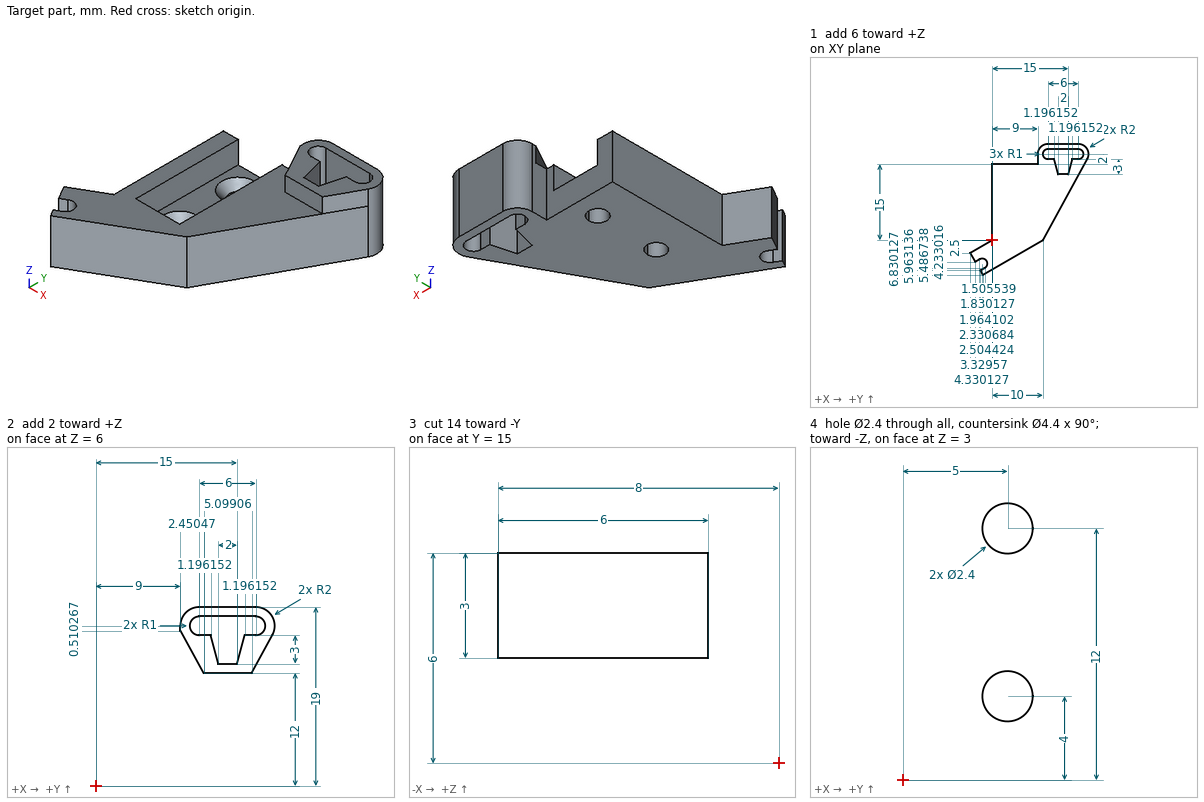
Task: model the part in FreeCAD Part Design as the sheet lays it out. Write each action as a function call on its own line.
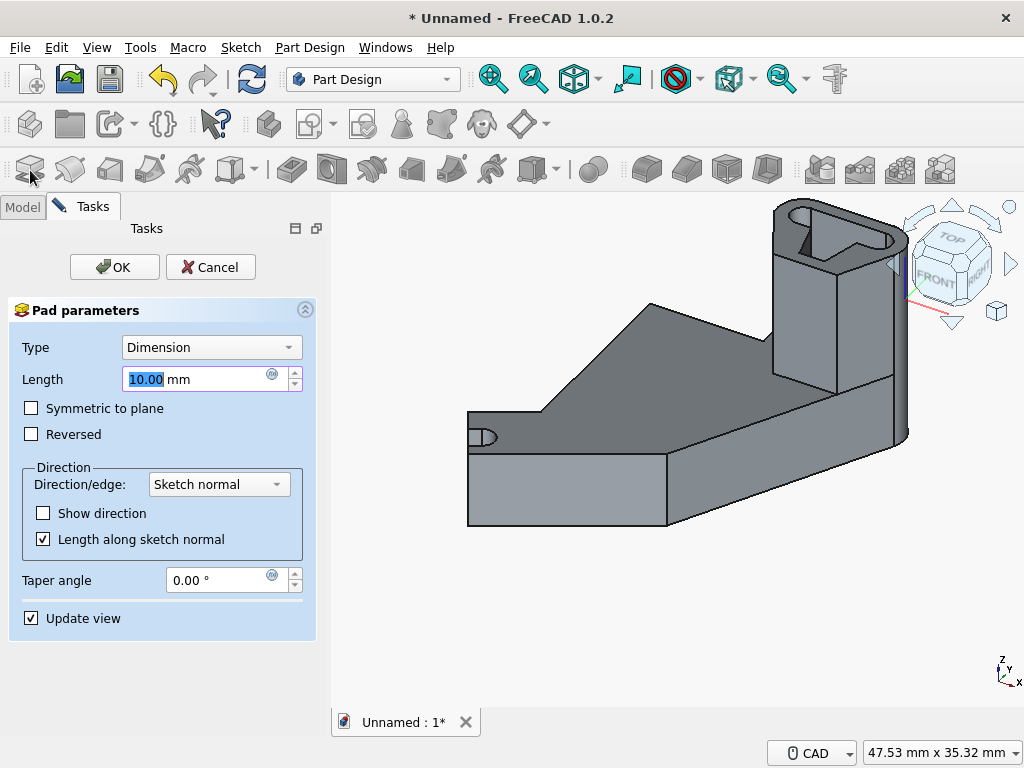
text(2)
key(Tab)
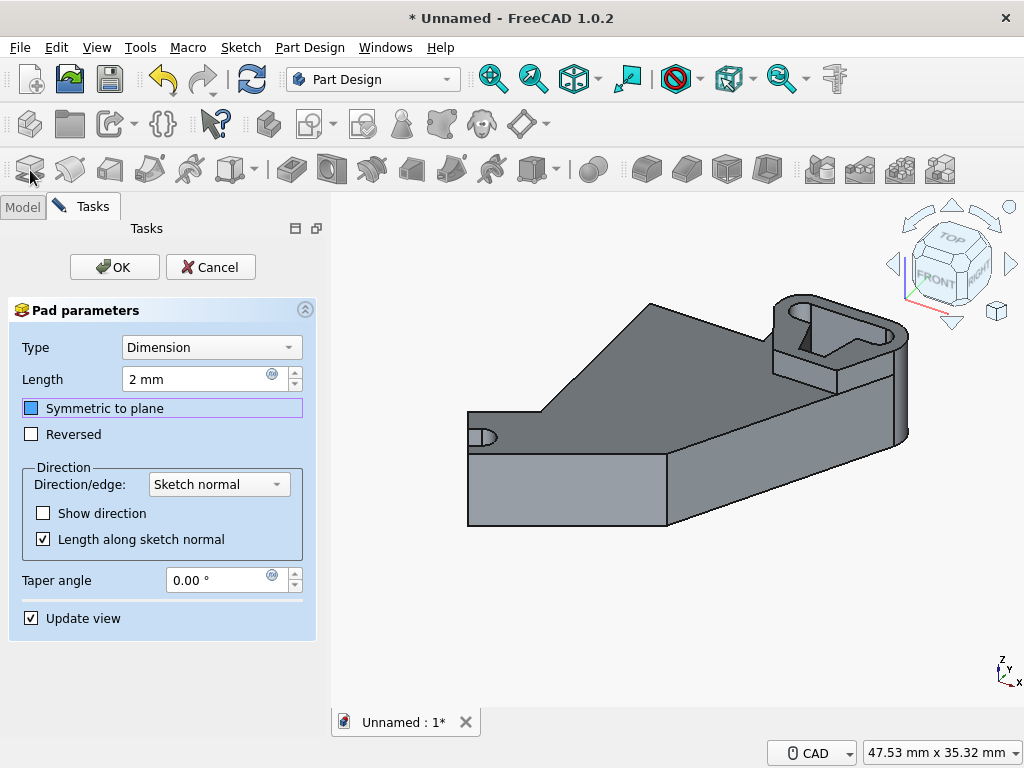
click(115, 267)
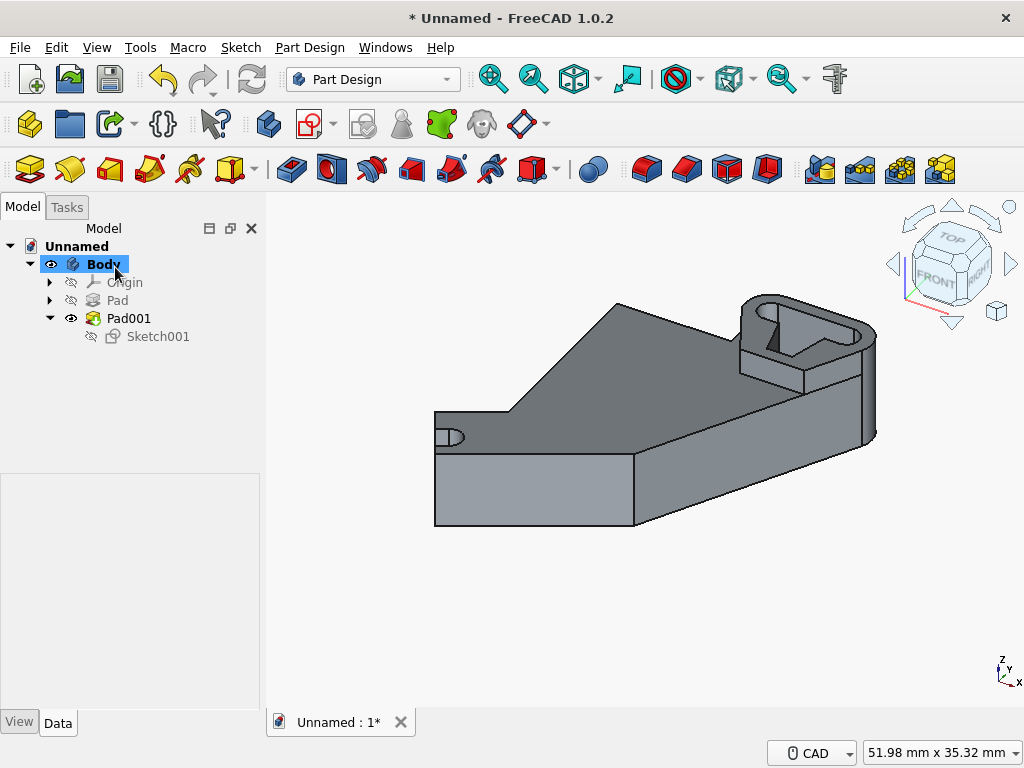
key(4)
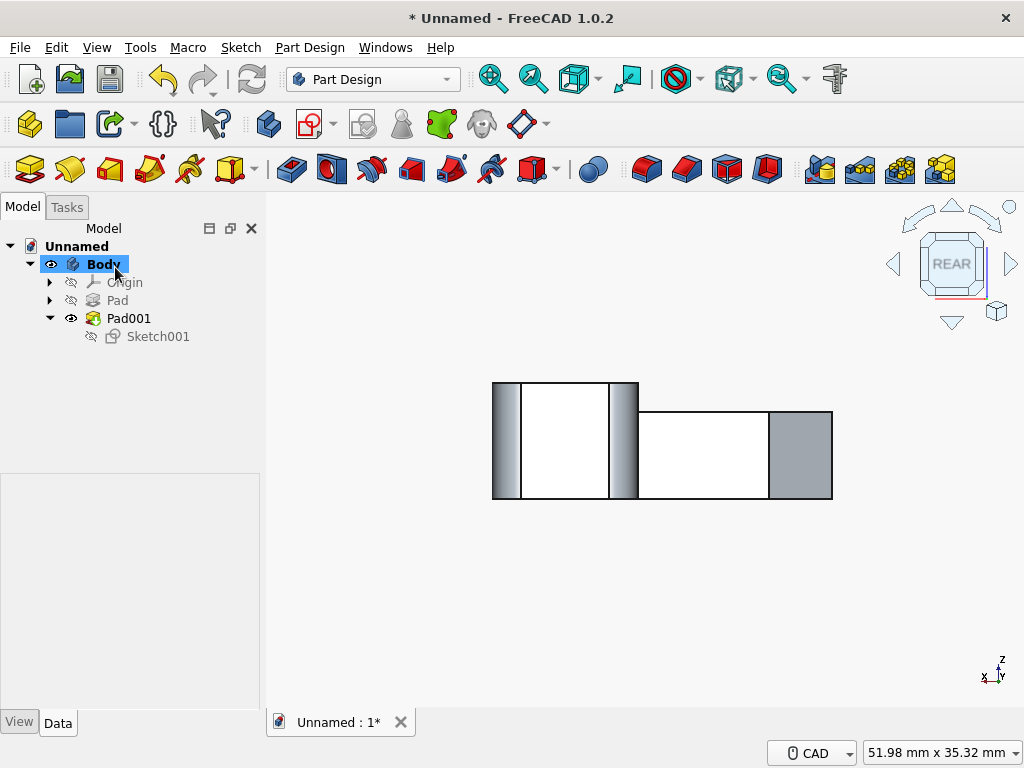
key(v)
key(f)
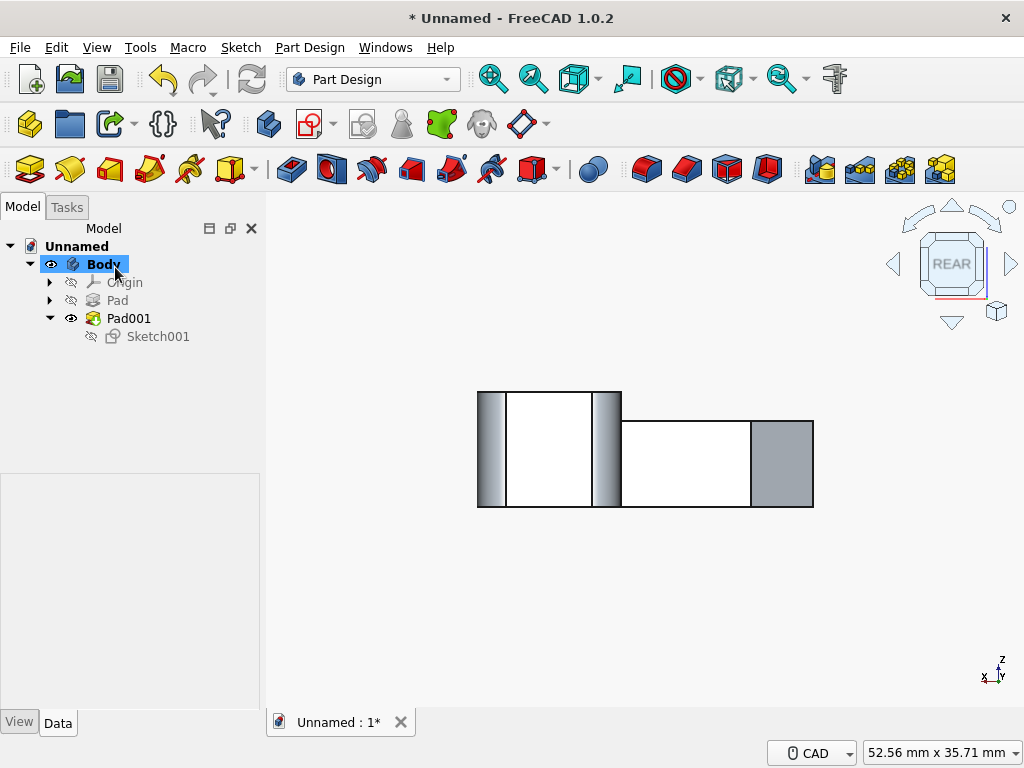
click(667, 463)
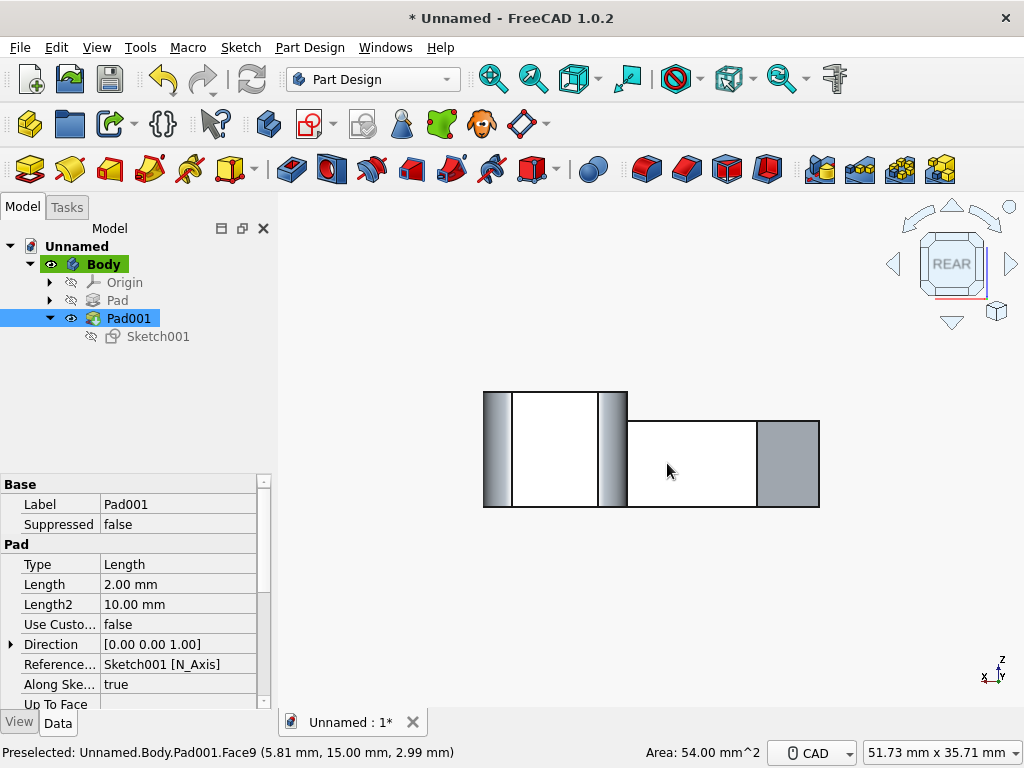
click(310, 124)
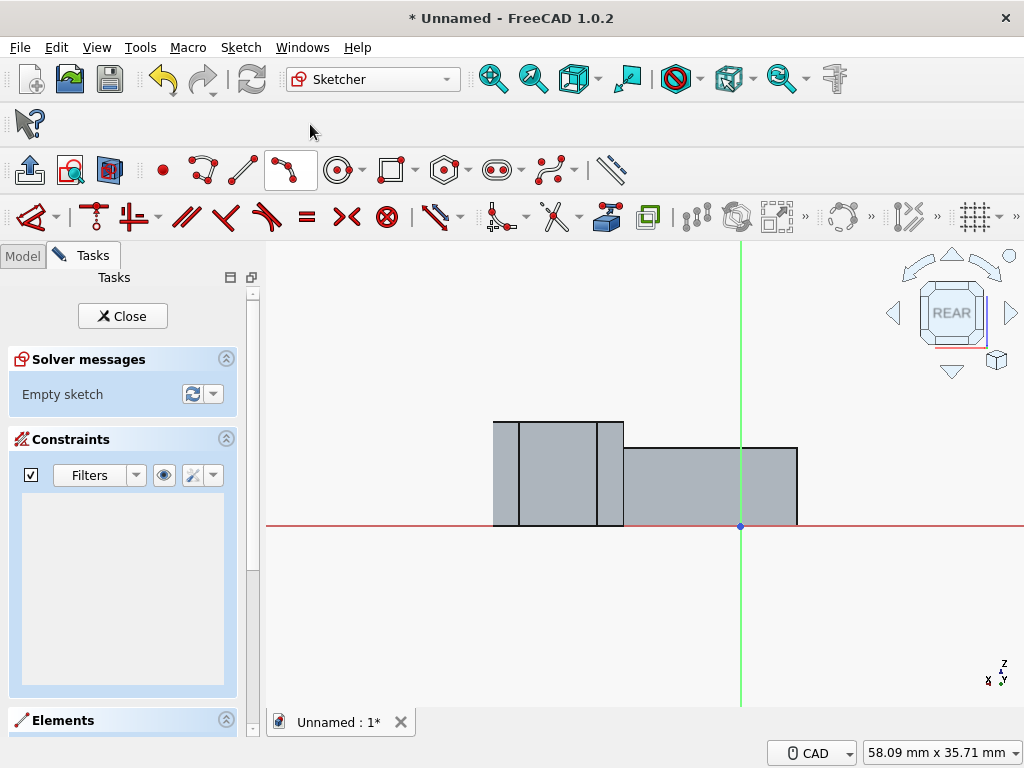
scroll(725, 491, up, 7)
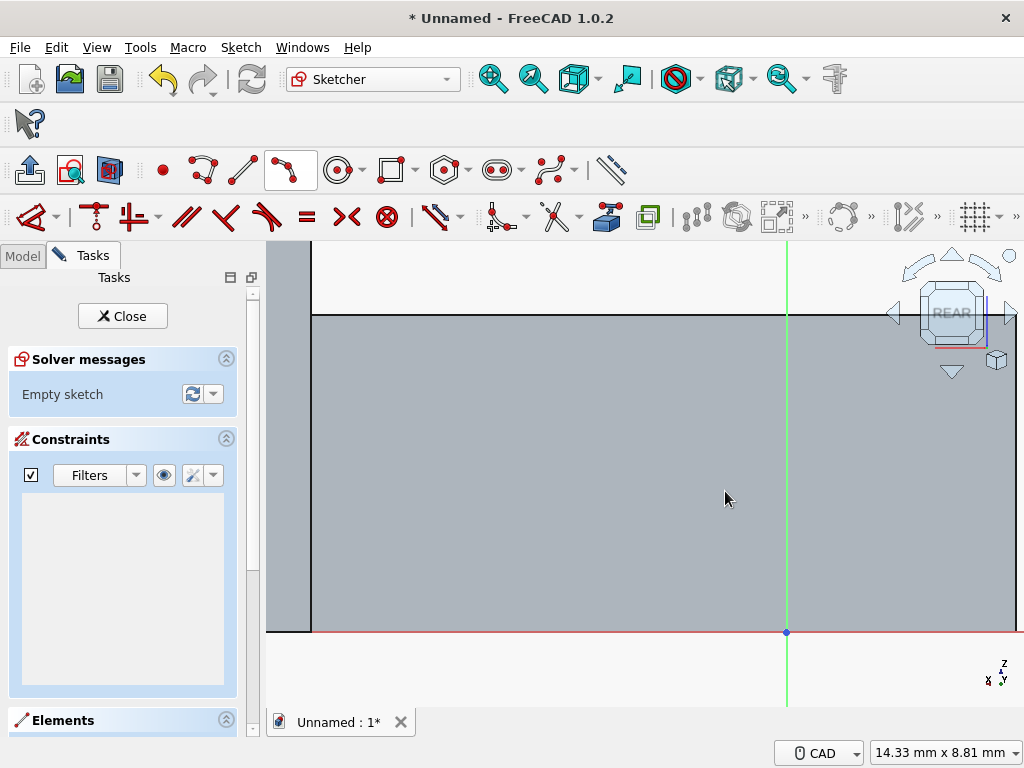
key(g)
key(r)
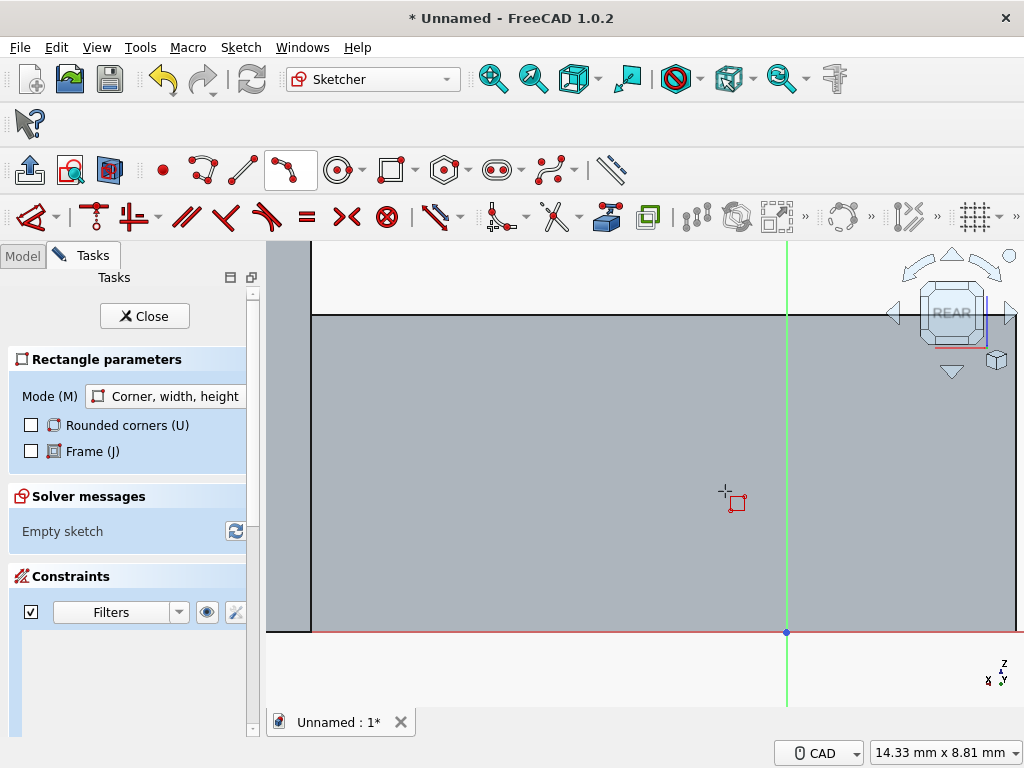
click(363, 315)
click(681, 473)
key(Escape)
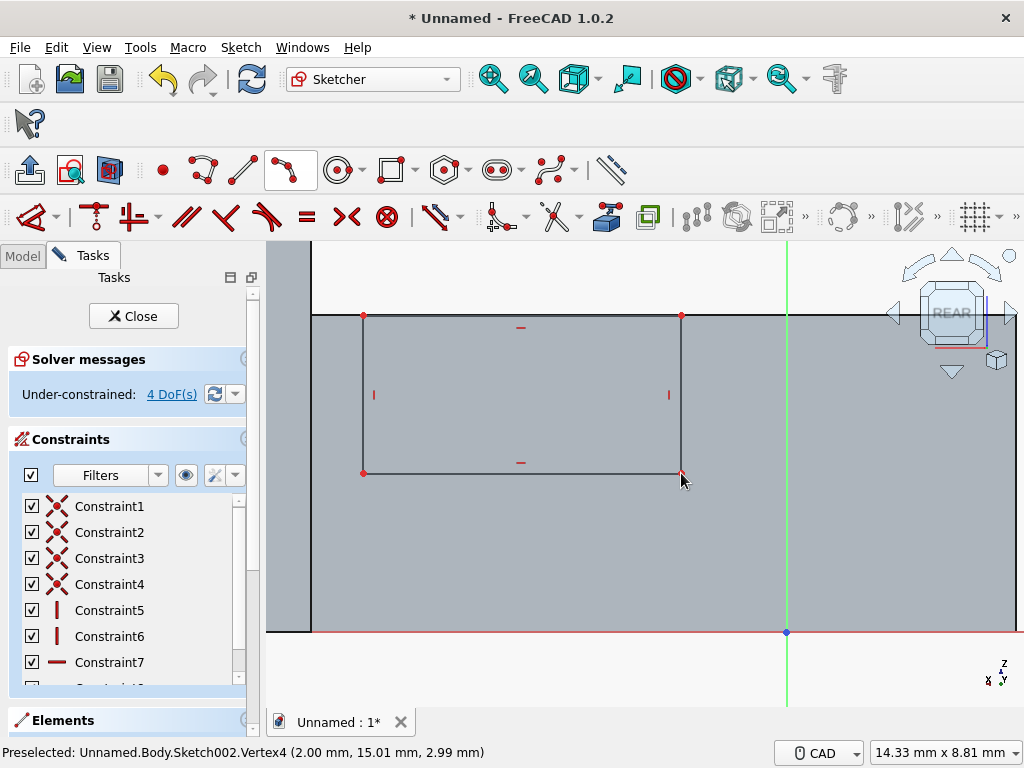
key(d)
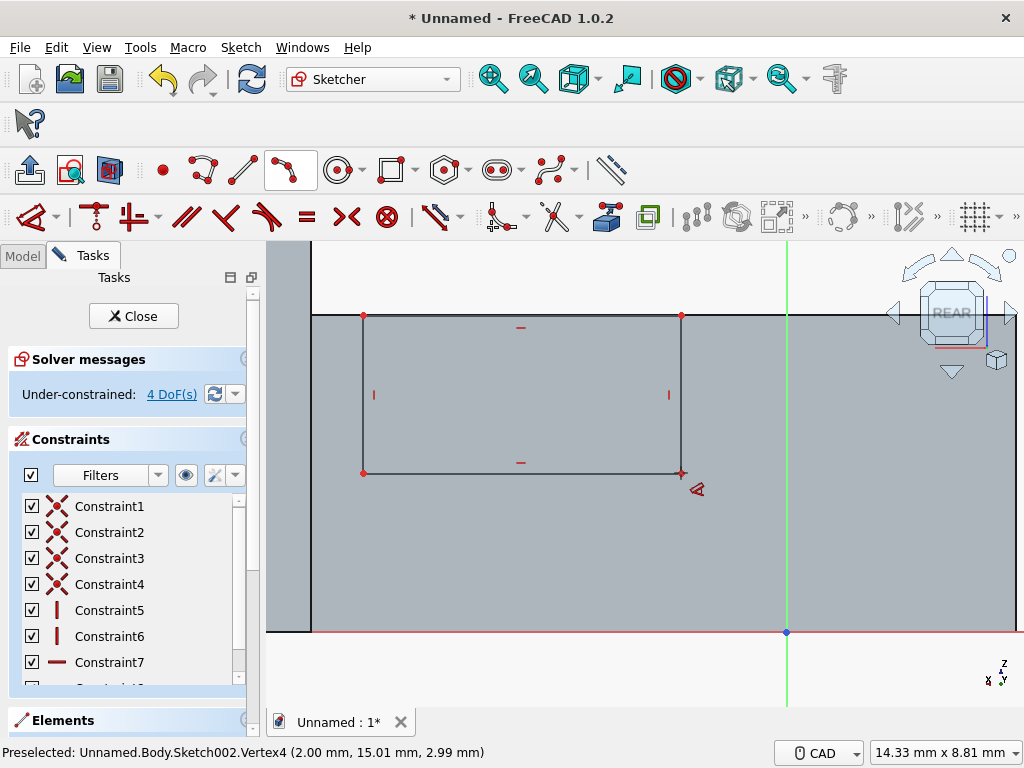
click(363, 363)
click(329, 395)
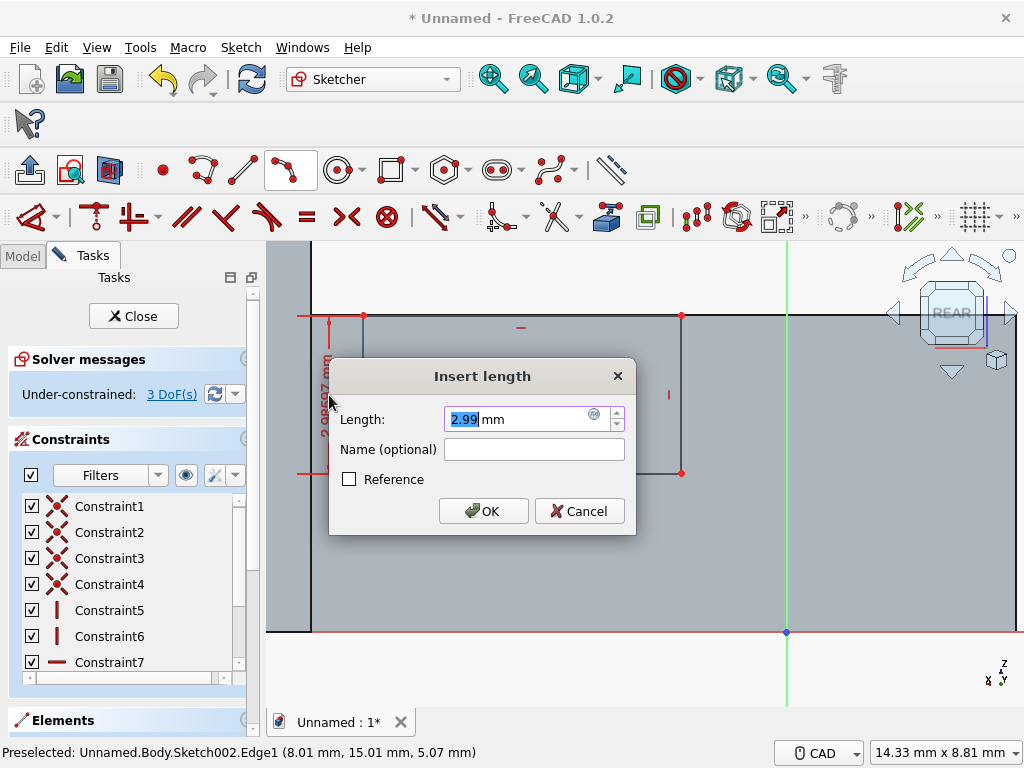
text(3)
key(Return)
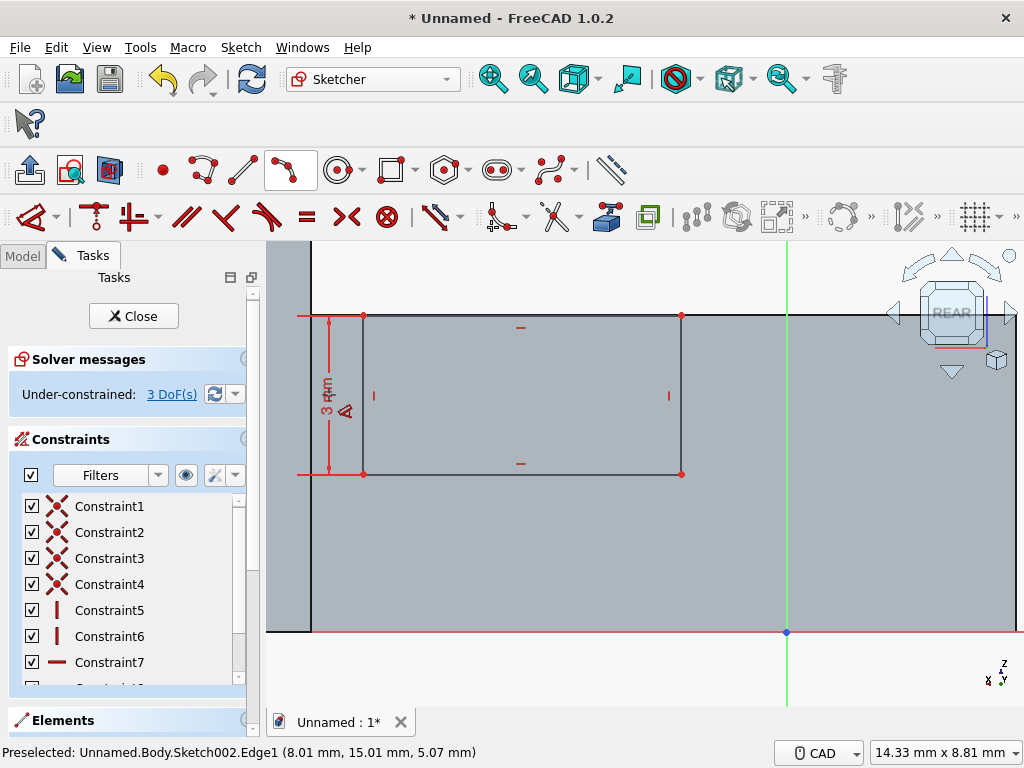
click(458, 475)
click(522, 509)